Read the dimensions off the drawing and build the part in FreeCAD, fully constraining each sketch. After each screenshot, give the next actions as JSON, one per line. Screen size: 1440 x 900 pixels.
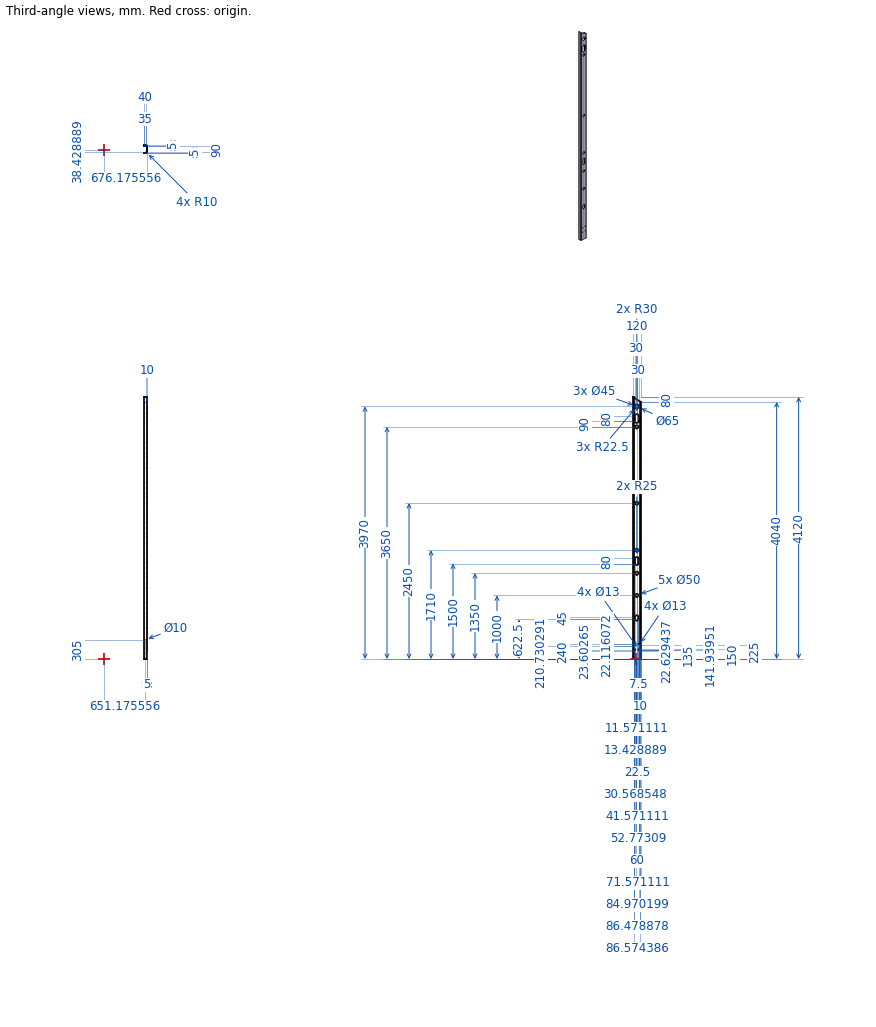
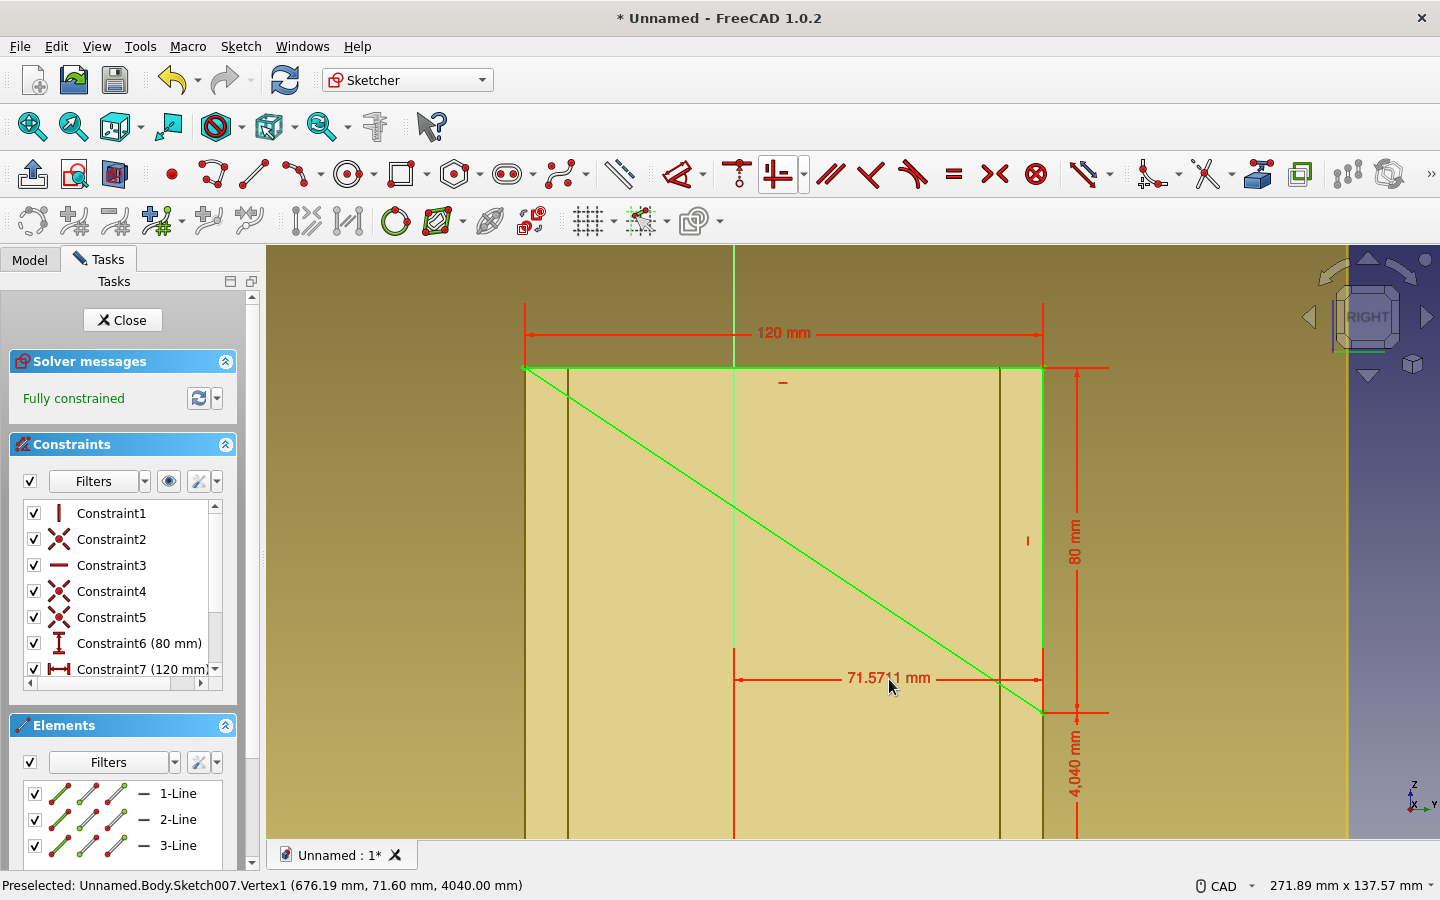
{"action": "left_click", "coordinate": [123, 320]}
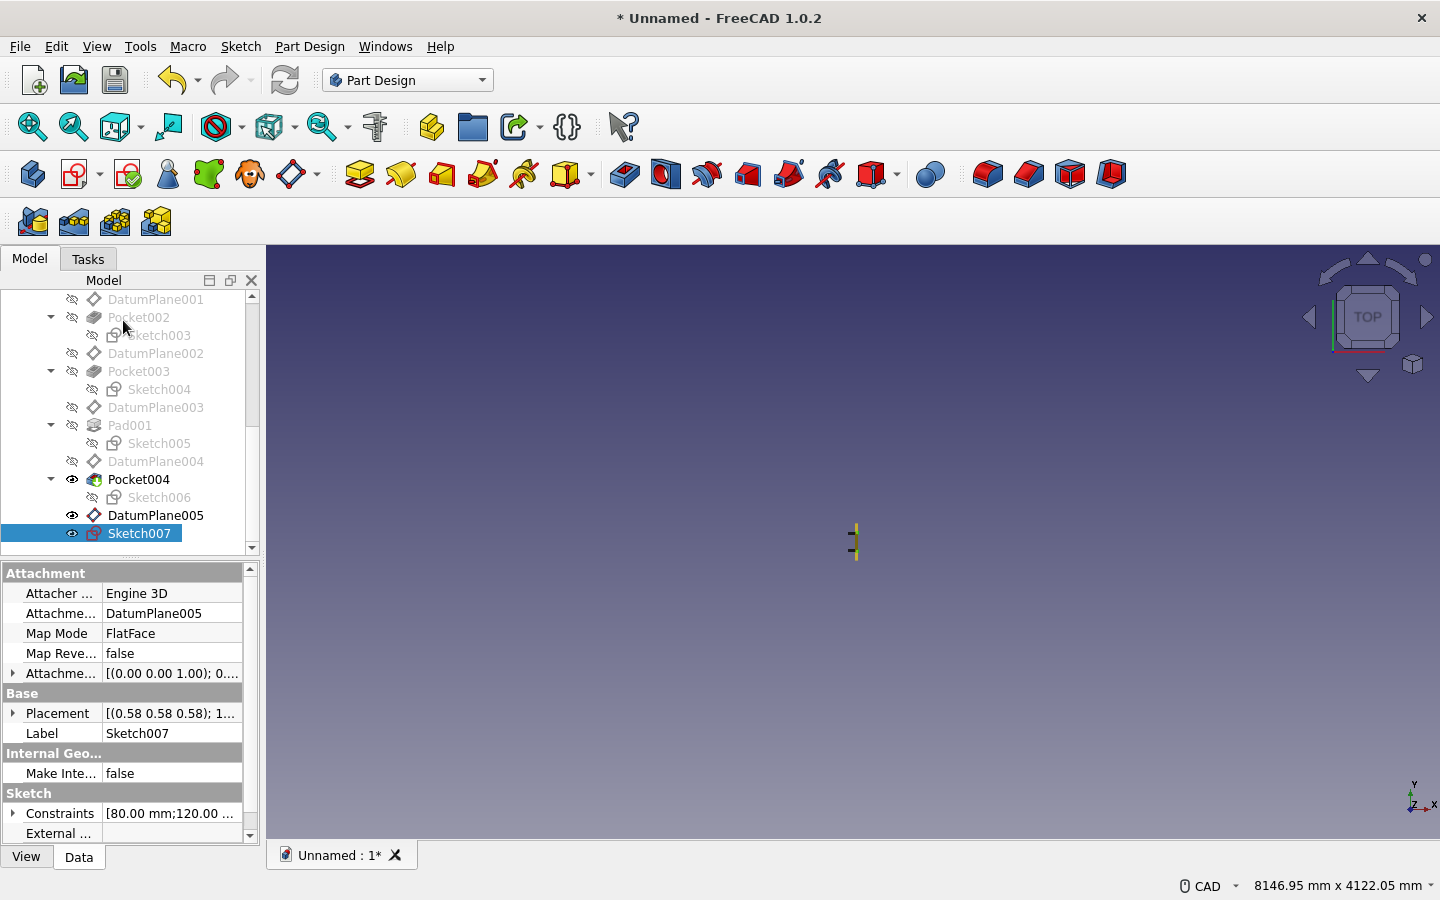
{"action": "left_click", "coordinate": [625, 174]}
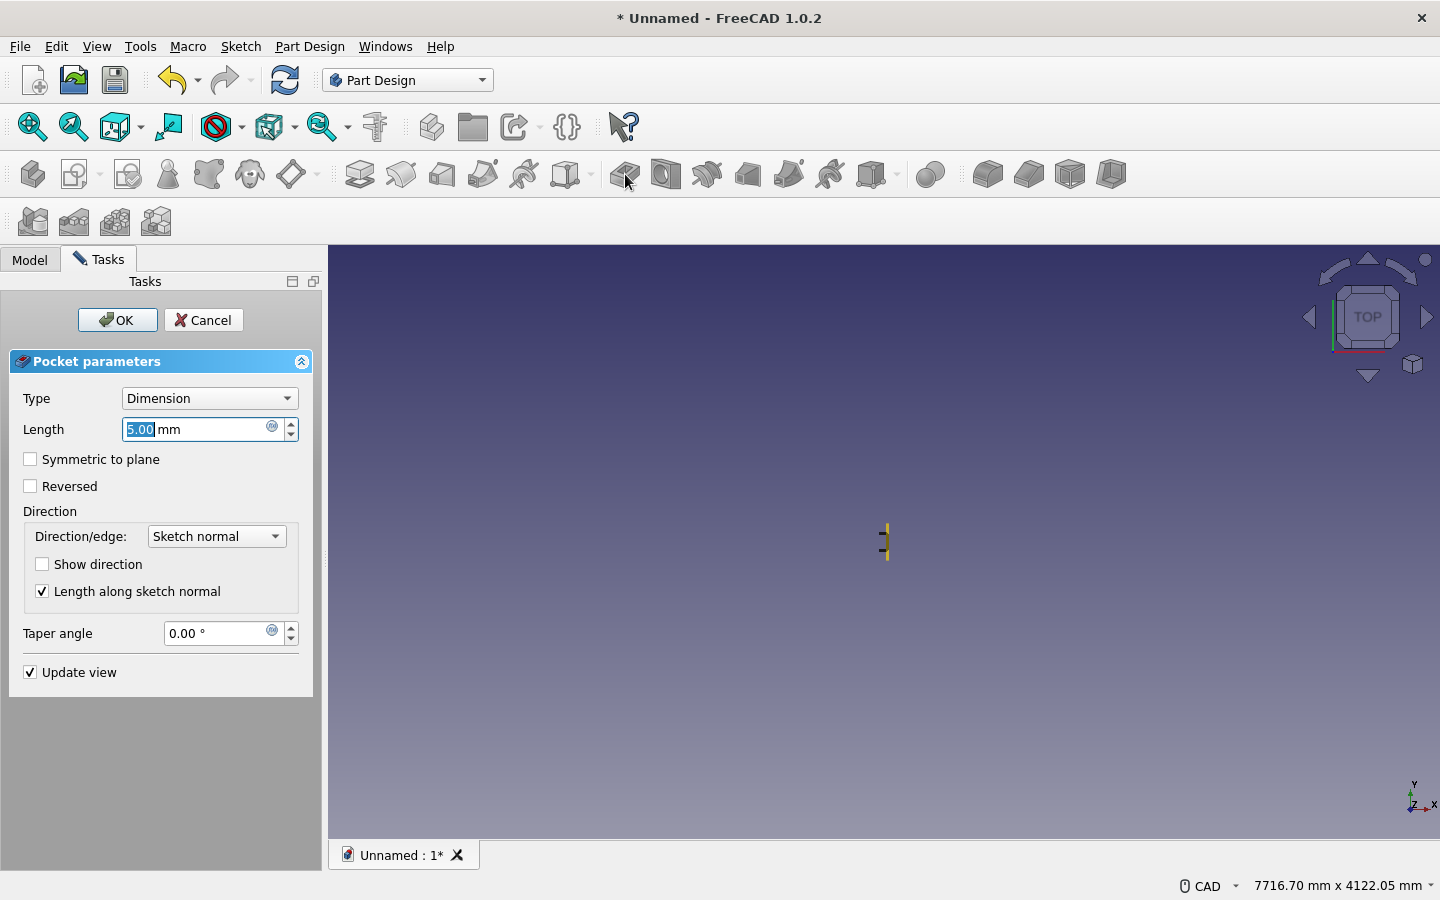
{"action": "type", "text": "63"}
{"action": "key", "text": "Tab"}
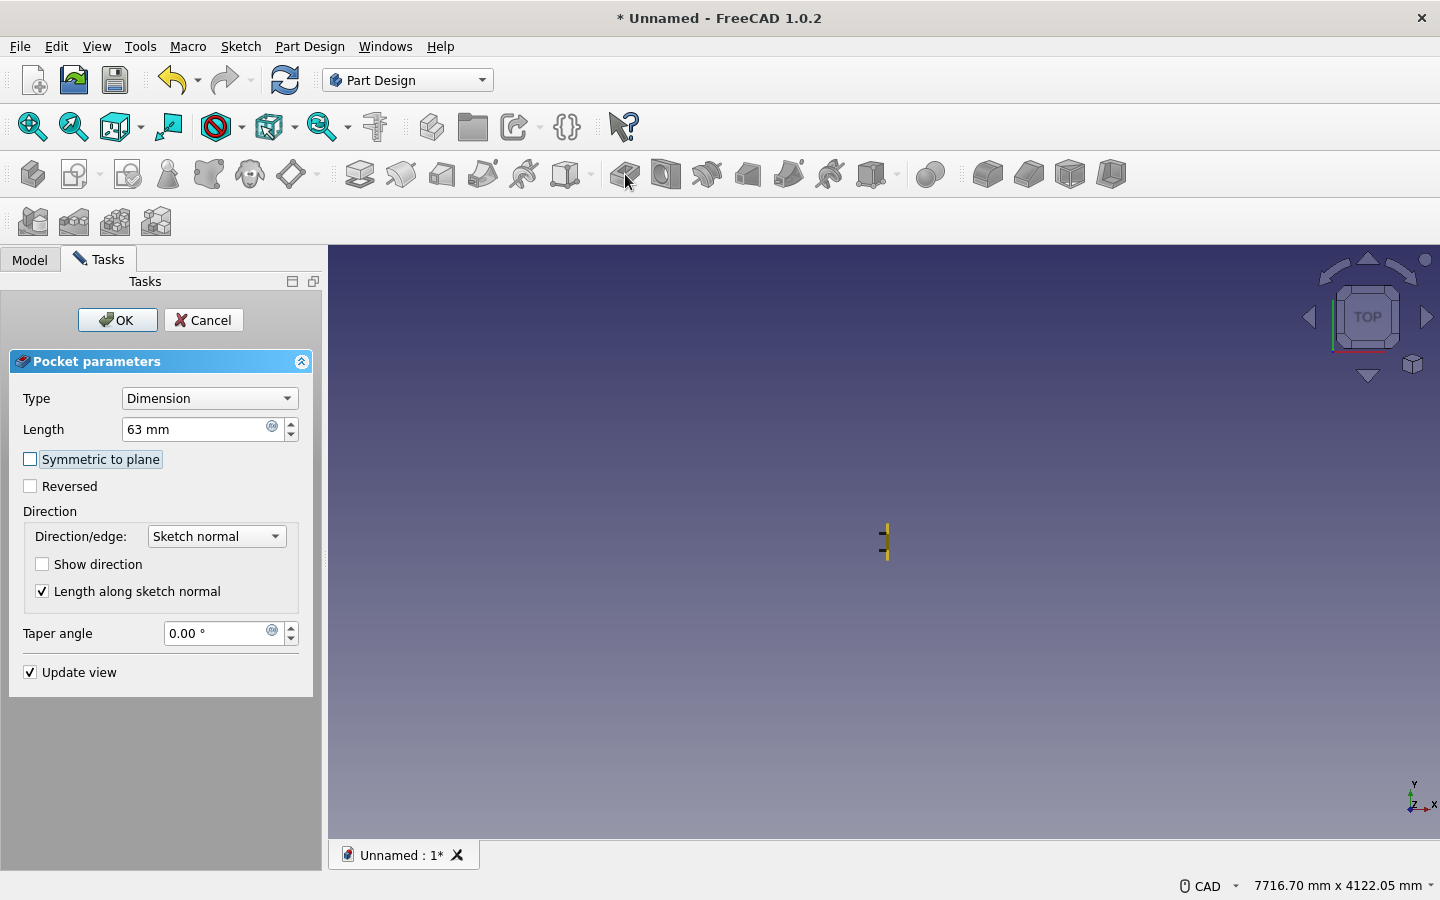
{"action": "left_click", "coordinate": [118, 320]}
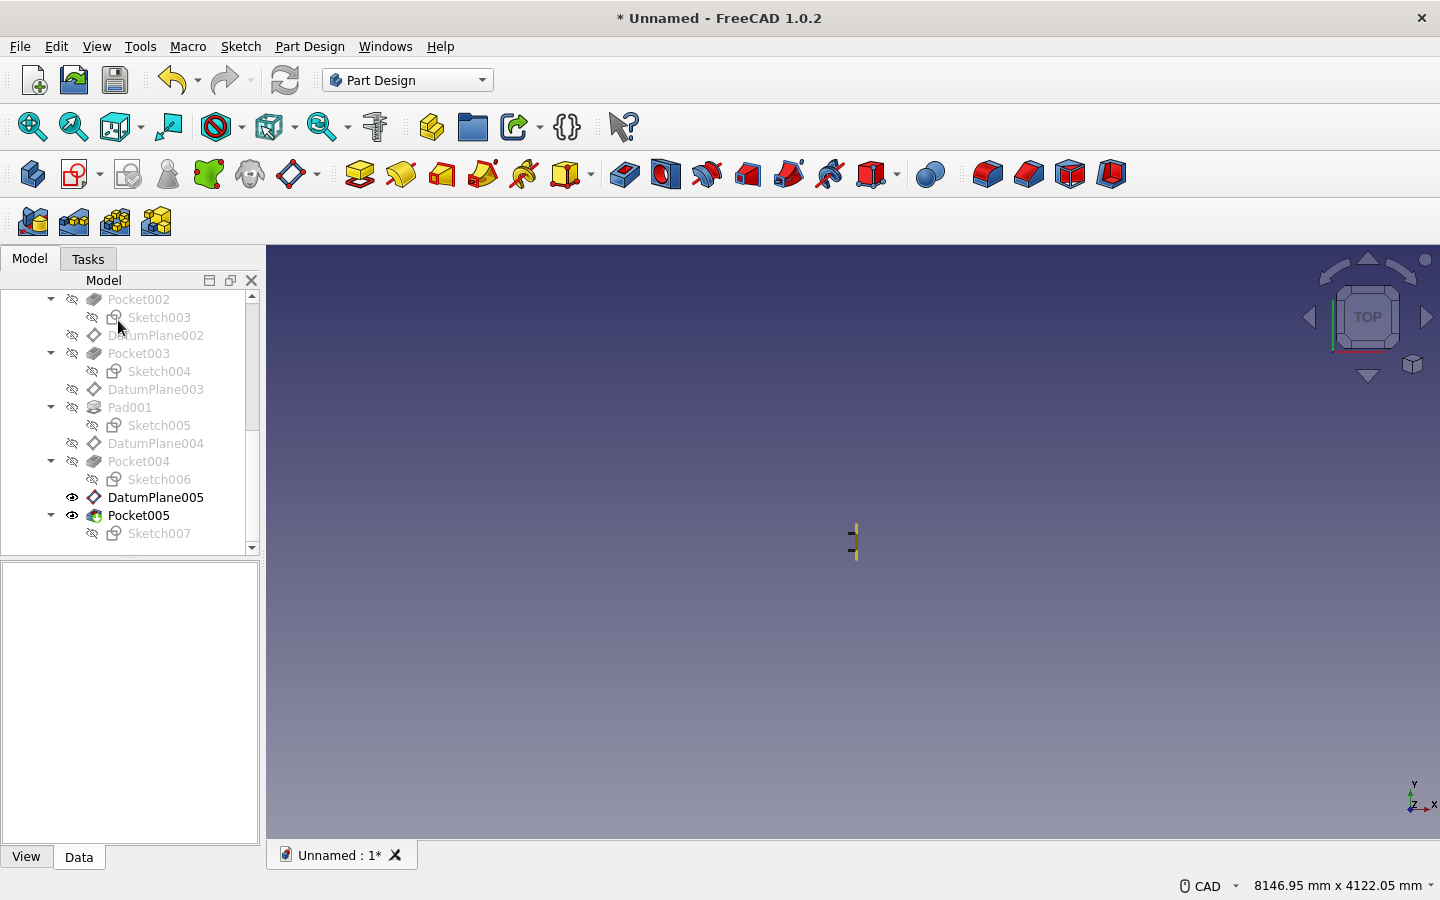
{"action": "left_click", "coordinate": [117, 497]}
{"action": "key", "text": "space"}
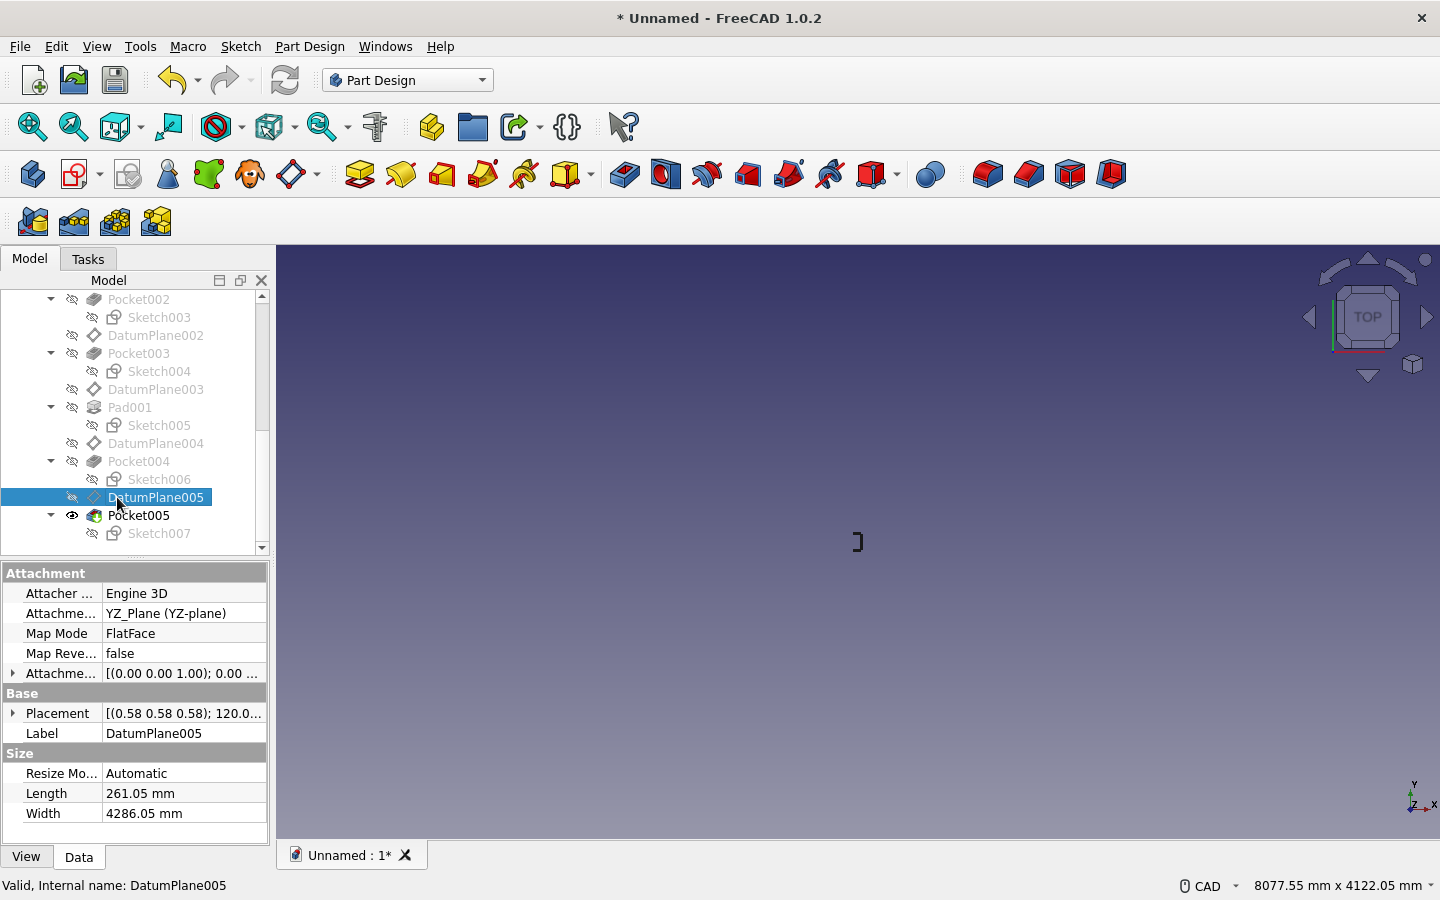
{"action": "key", "text": "0"}